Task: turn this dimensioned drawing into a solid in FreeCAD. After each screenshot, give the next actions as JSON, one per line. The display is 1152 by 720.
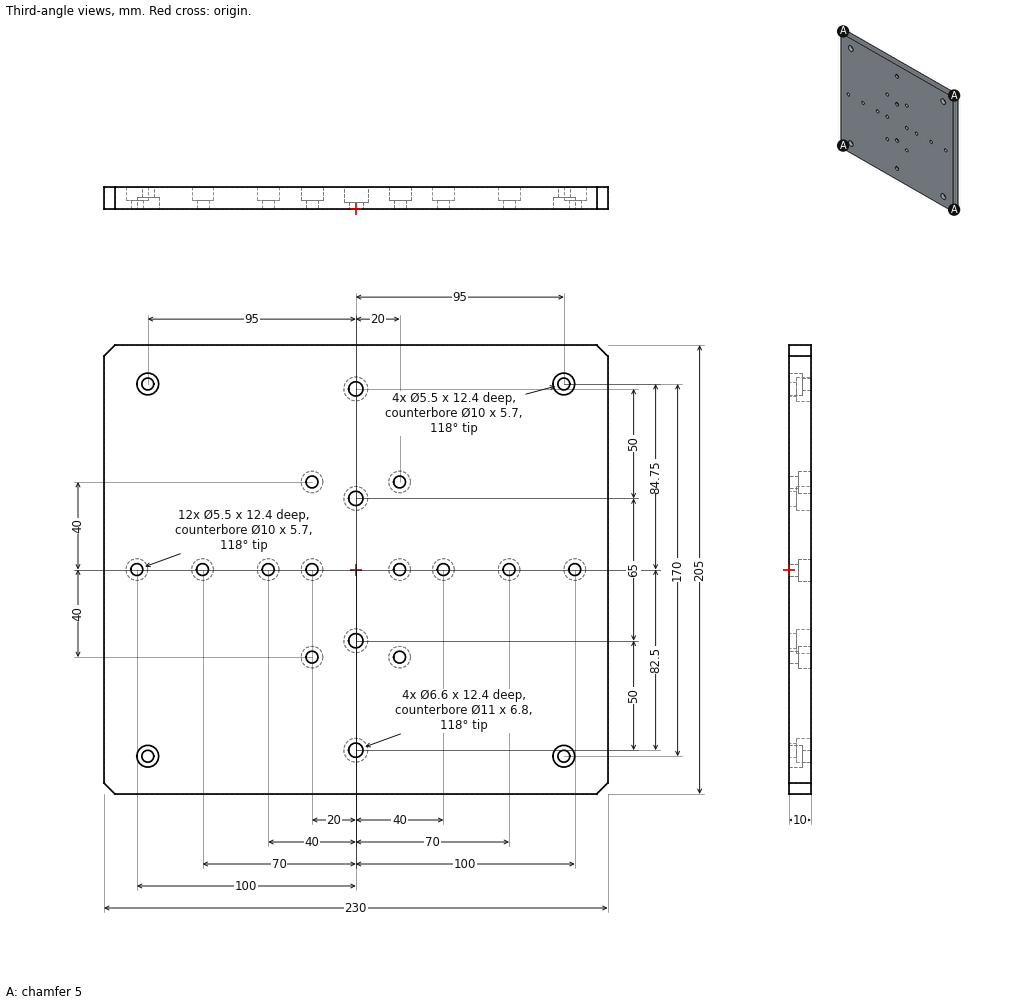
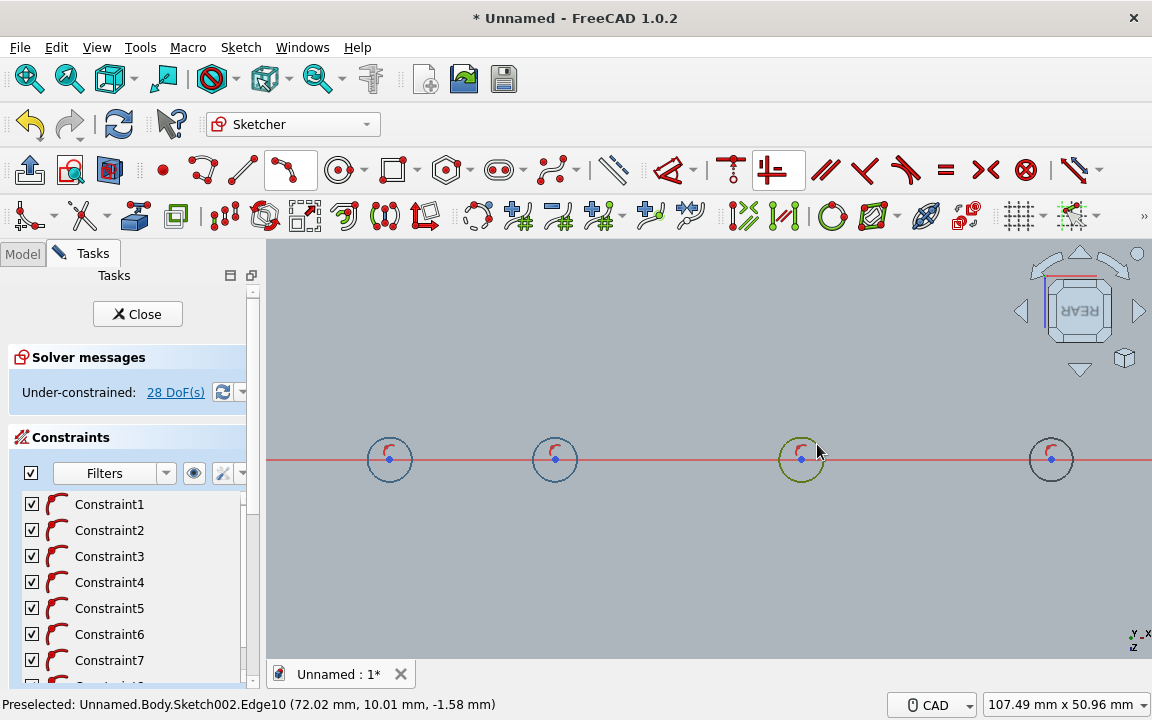
{"action": "scroll", "coordinate": [819, 444], "scroll_direction": "down", "scroll_amount": 6}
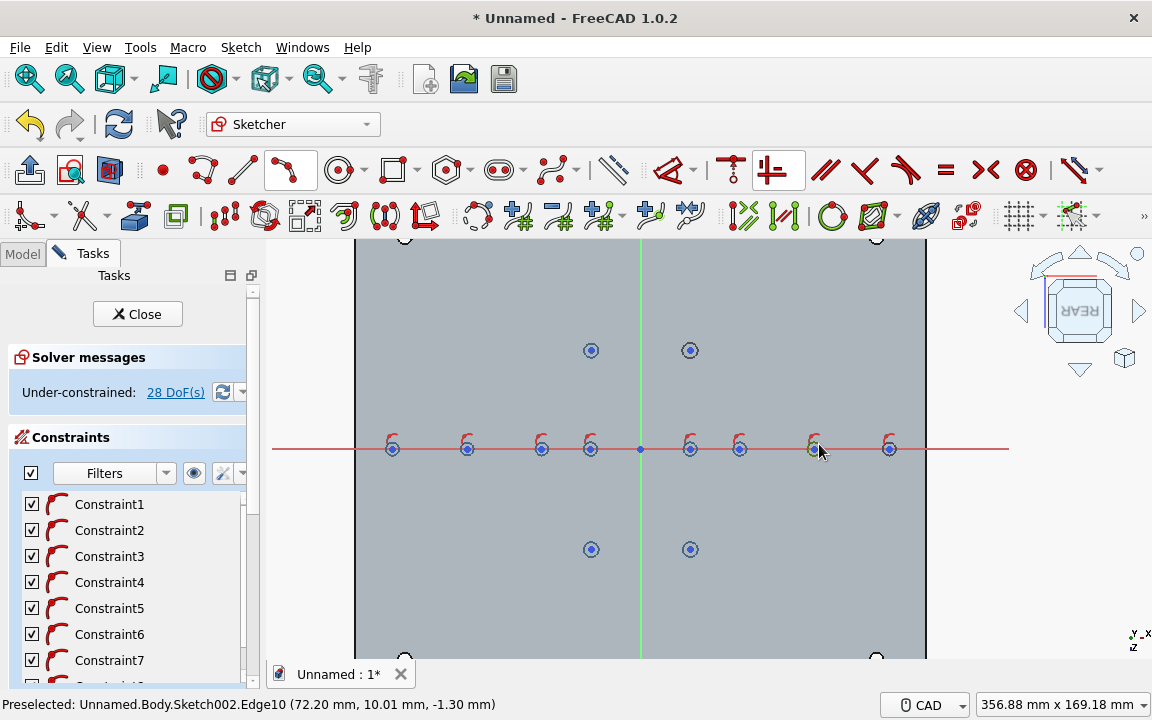
{"action": "scroll", "coordinate": [894, 444], "scroll_direction": "up", "scroll_amount": 6}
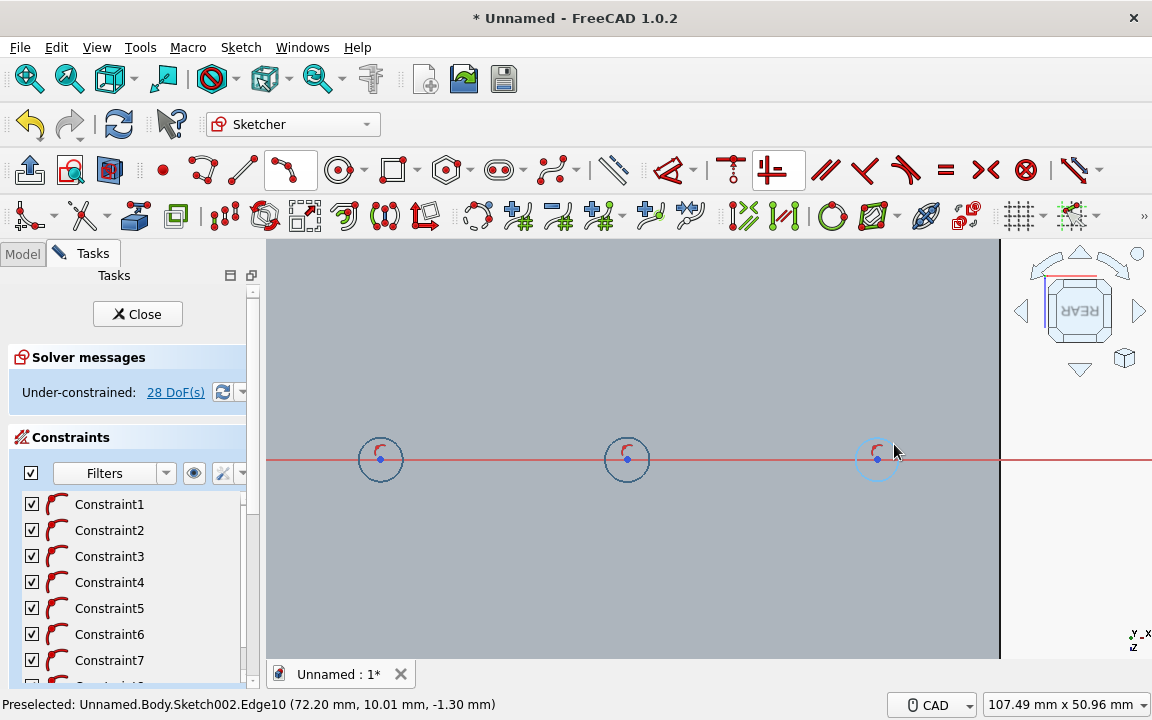
{"action": "left_click", "coordinate": [892, 444]}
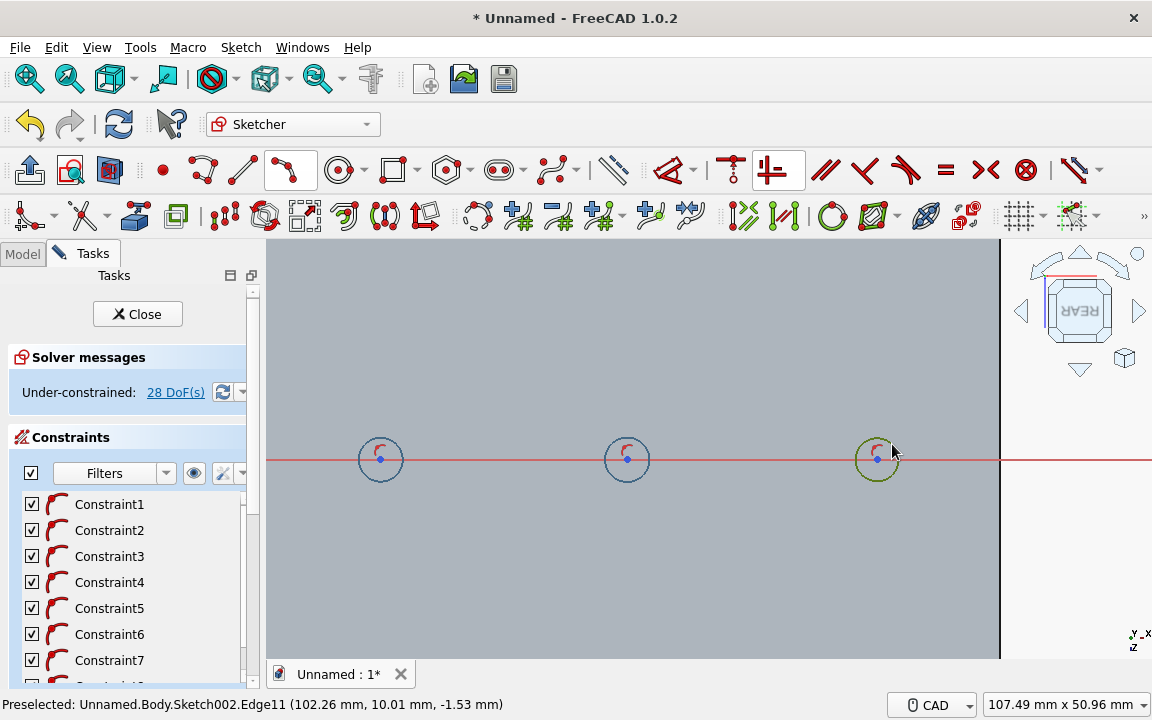
{"action": "scroll", "coordinate": [894, 444], "scroll_direction": "down", "scroll_amount": 6}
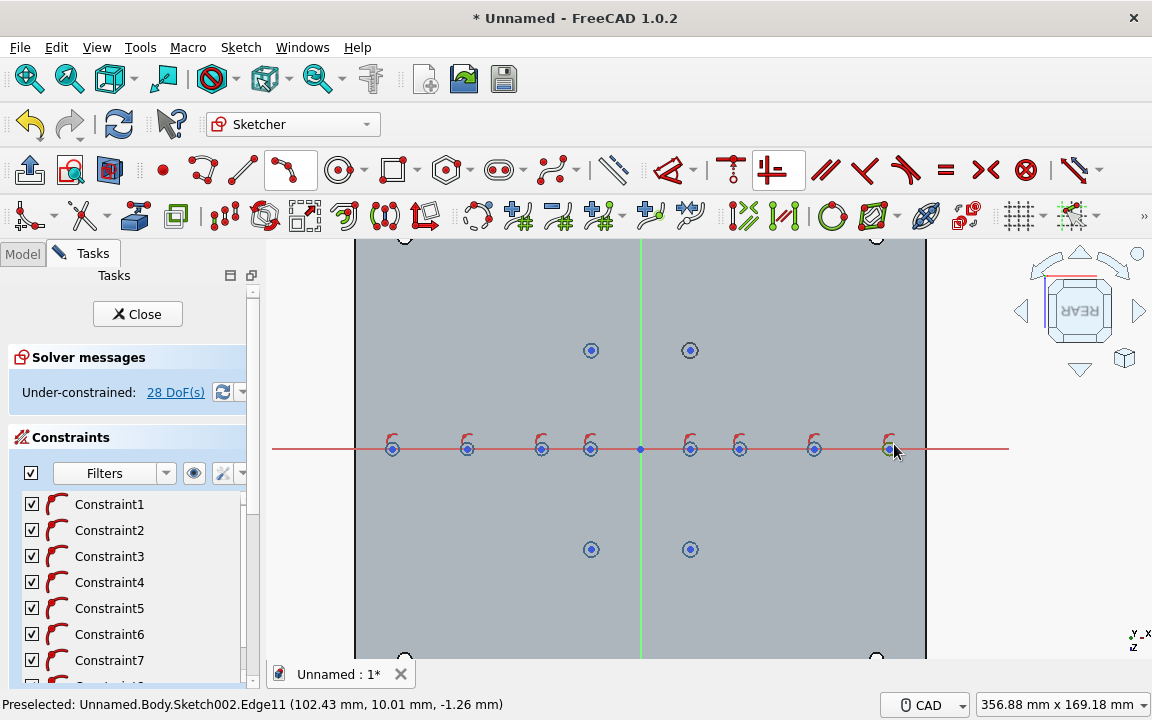
{"action": "scroll", "coordinate": [695, 345], "scroll_direction": "up", "scroll_amount": 3}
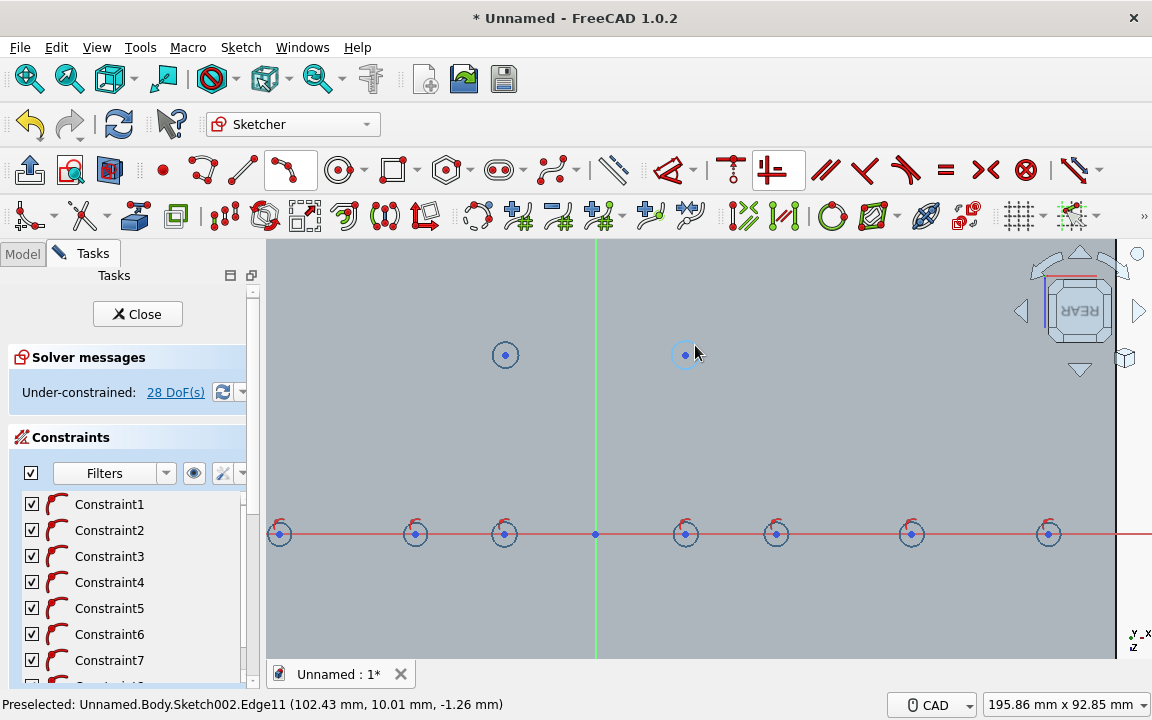
{"action": "left_click", "coordinate": [695, 345]}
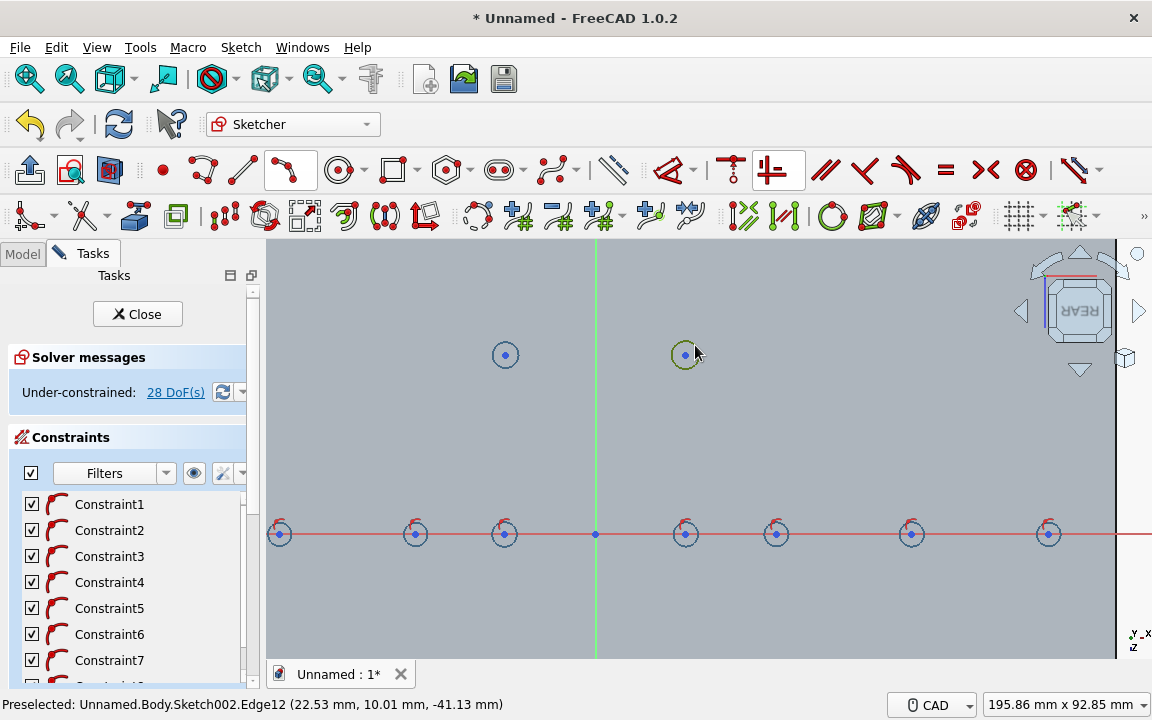
{"action": "left_click", "coordinate": [946, 170]}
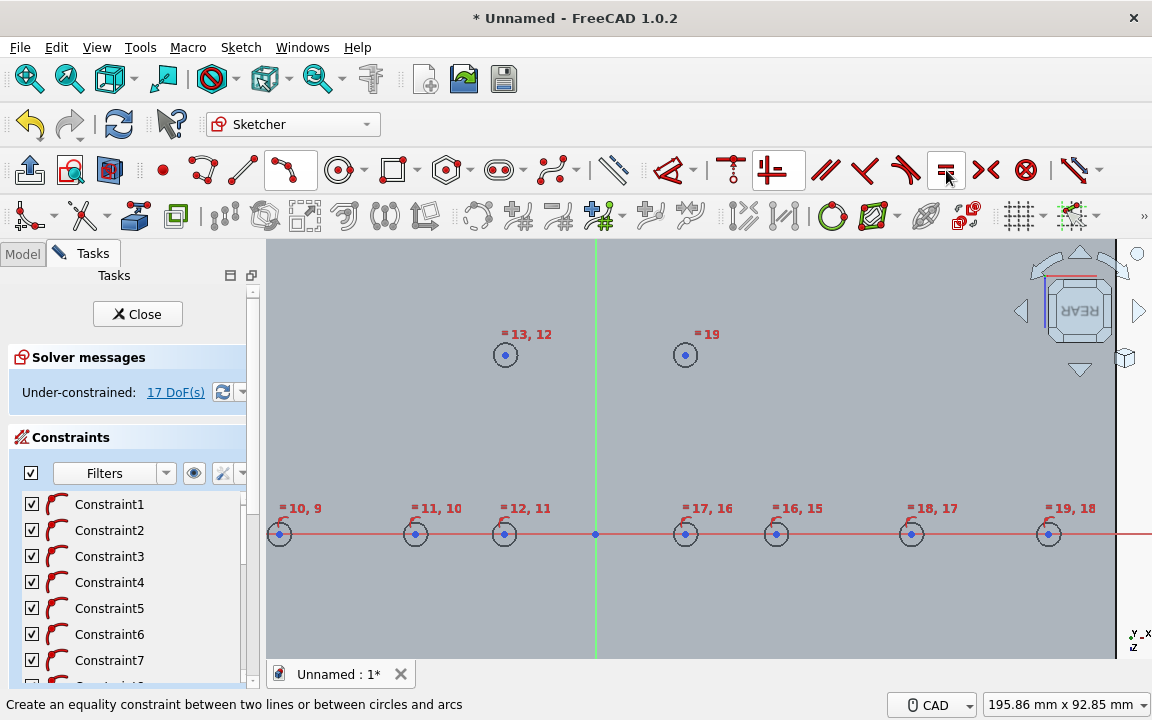
{"action": "left_click", "coordinate": [504, 534]}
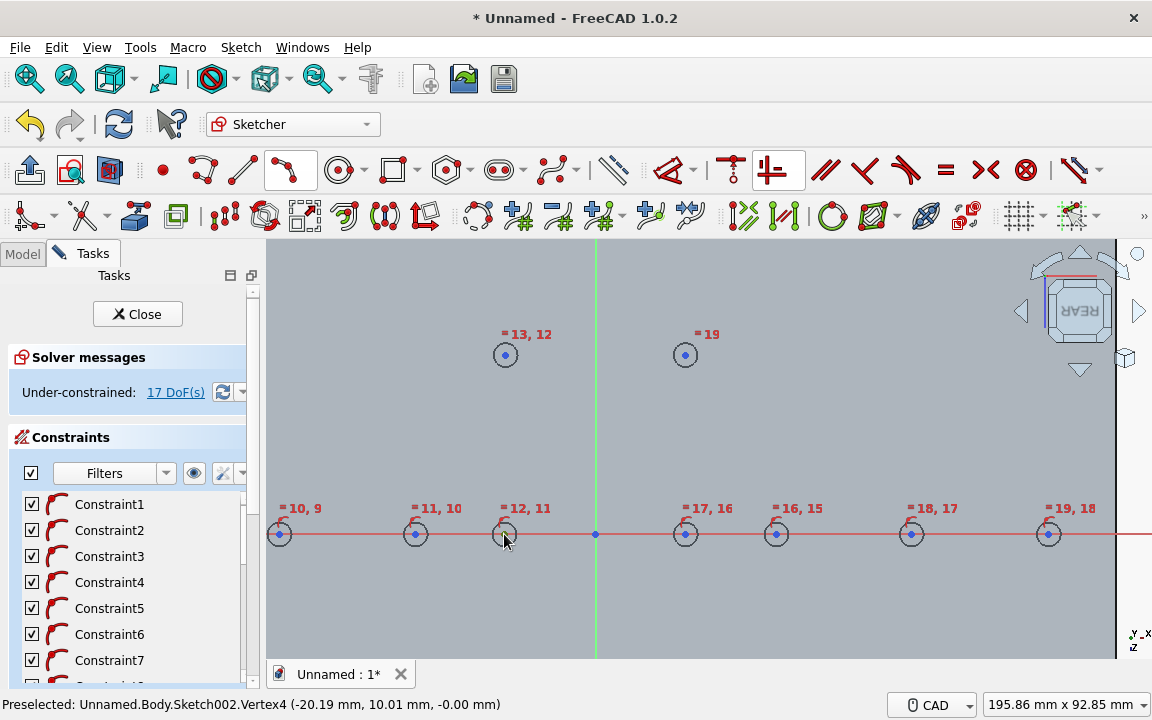
{"action": "left_click", "coordinate": [506, 355]}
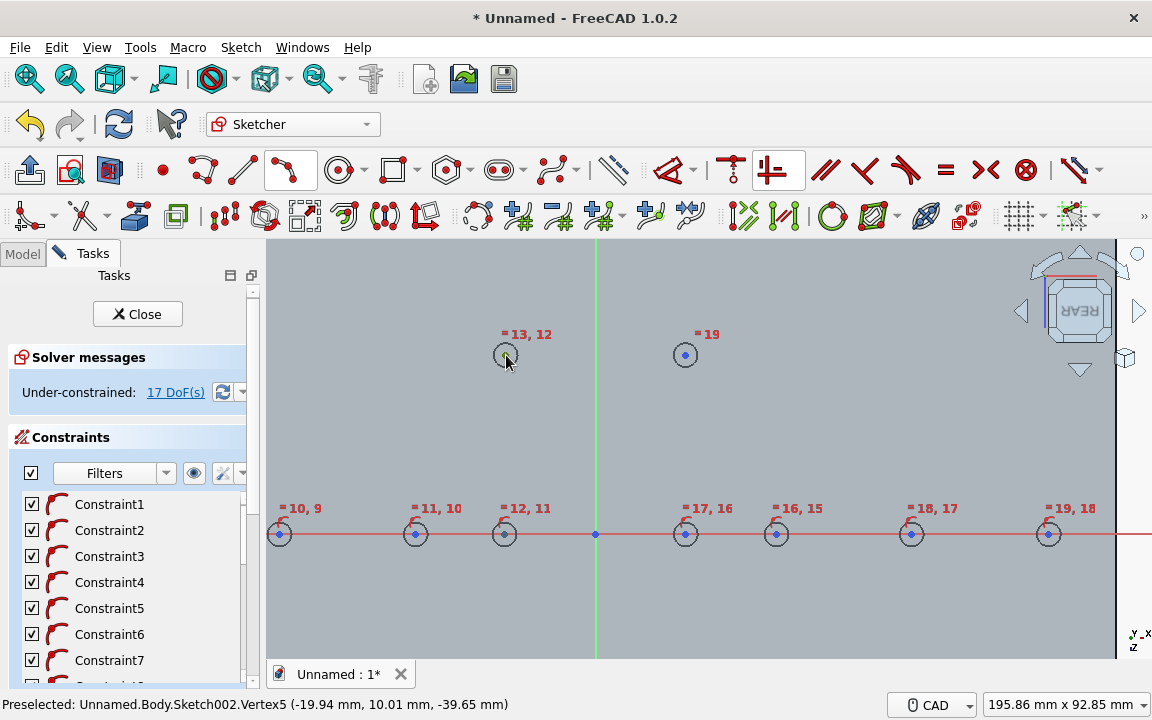
{"action": "left_click", "coordinate": [800, 170]}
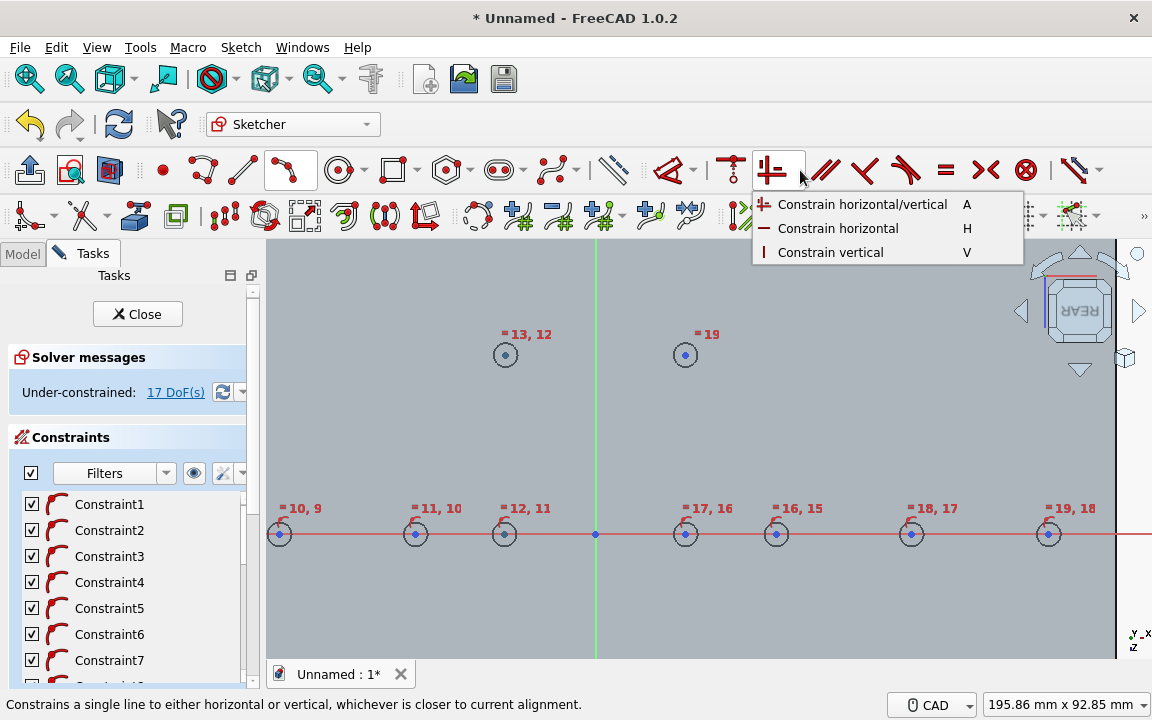
{"action": "left_click", "coordinate": [888, 252]}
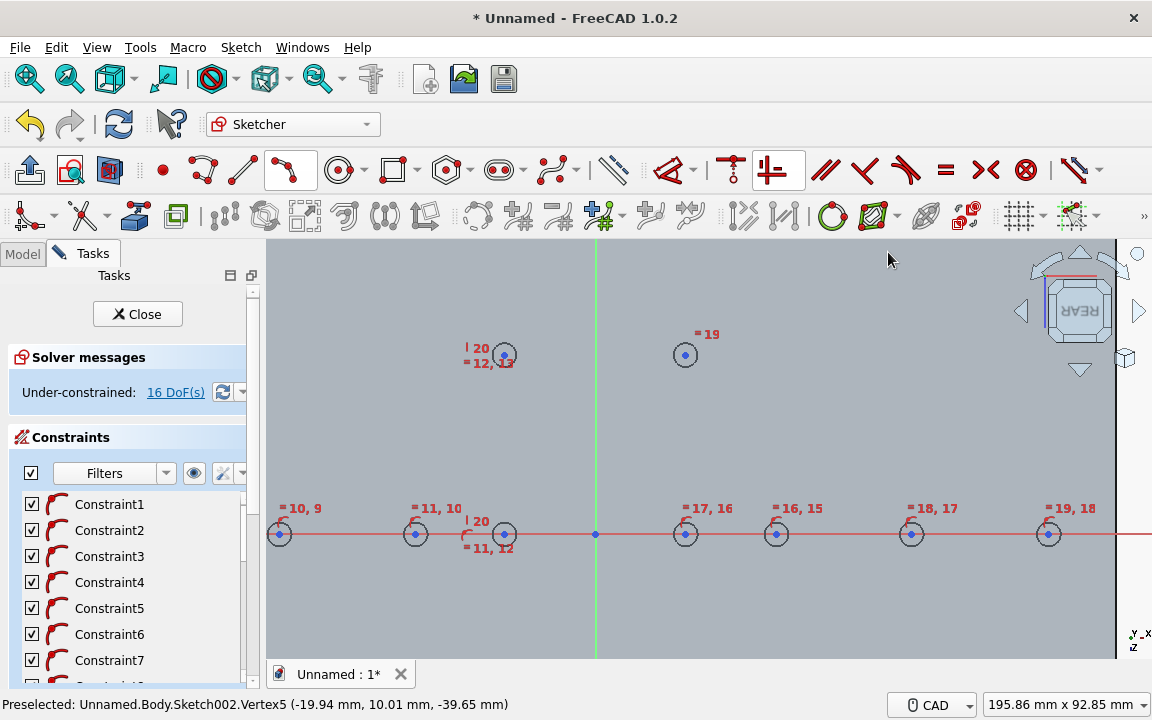
{"action": "left_click", "coordinate": [504, 534]}